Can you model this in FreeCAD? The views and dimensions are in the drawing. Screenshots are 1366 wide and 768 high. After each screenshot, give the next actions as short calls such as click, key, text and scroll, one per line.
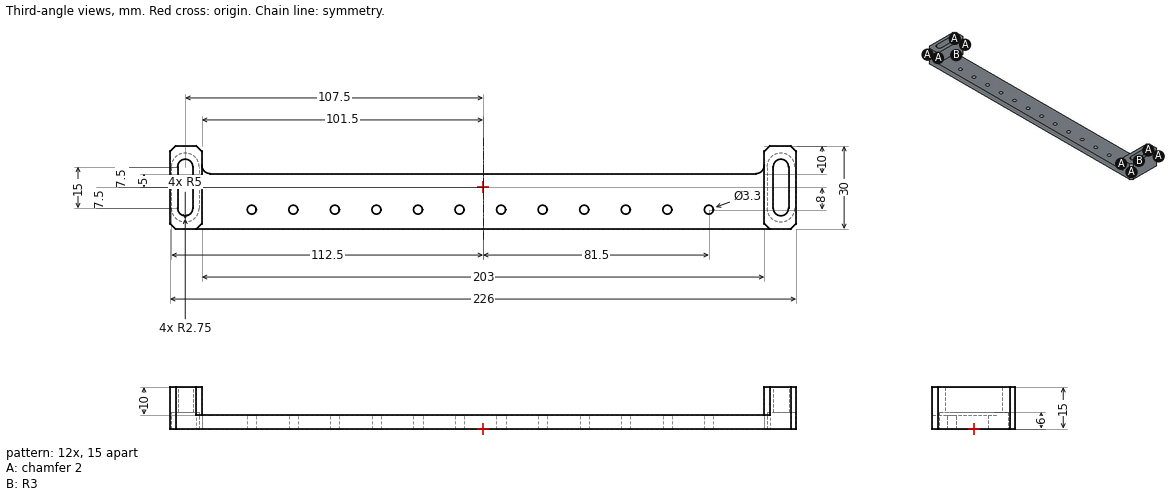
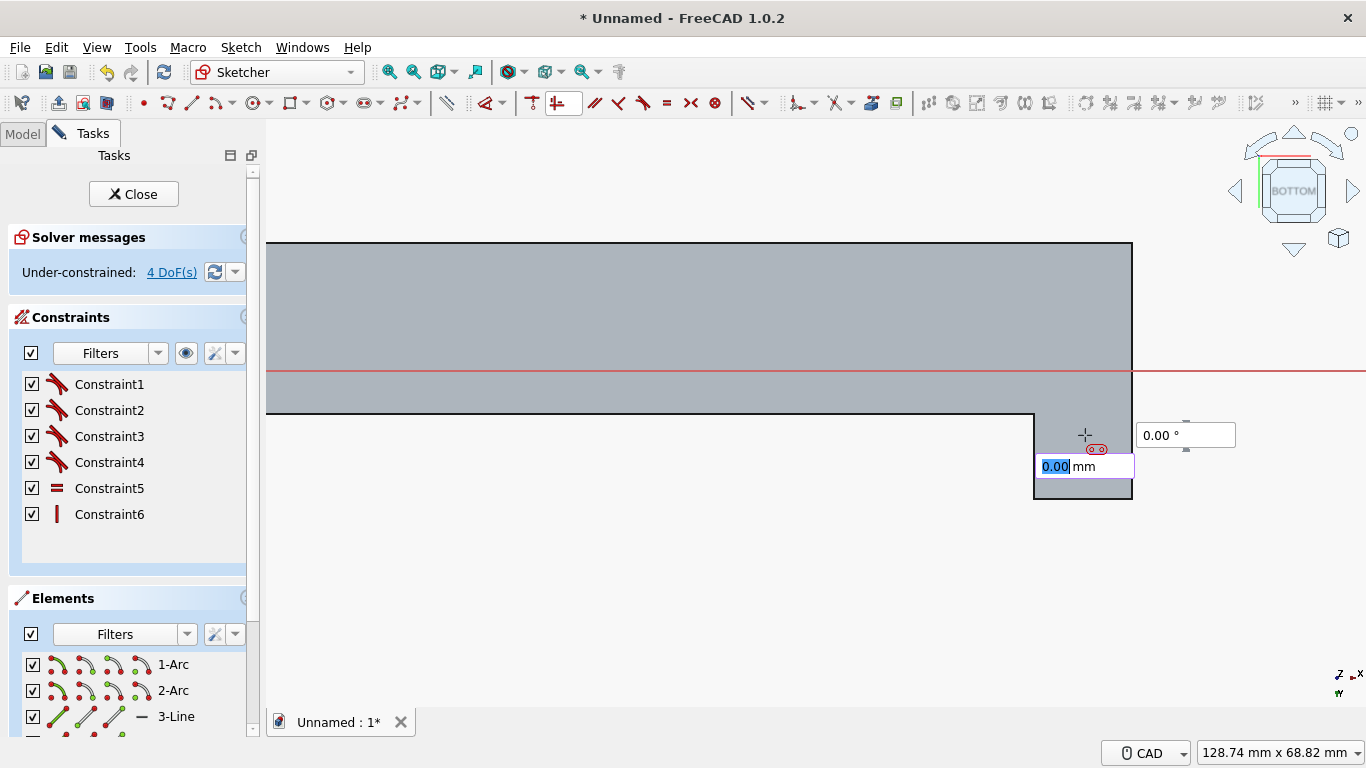
click(1085, 307)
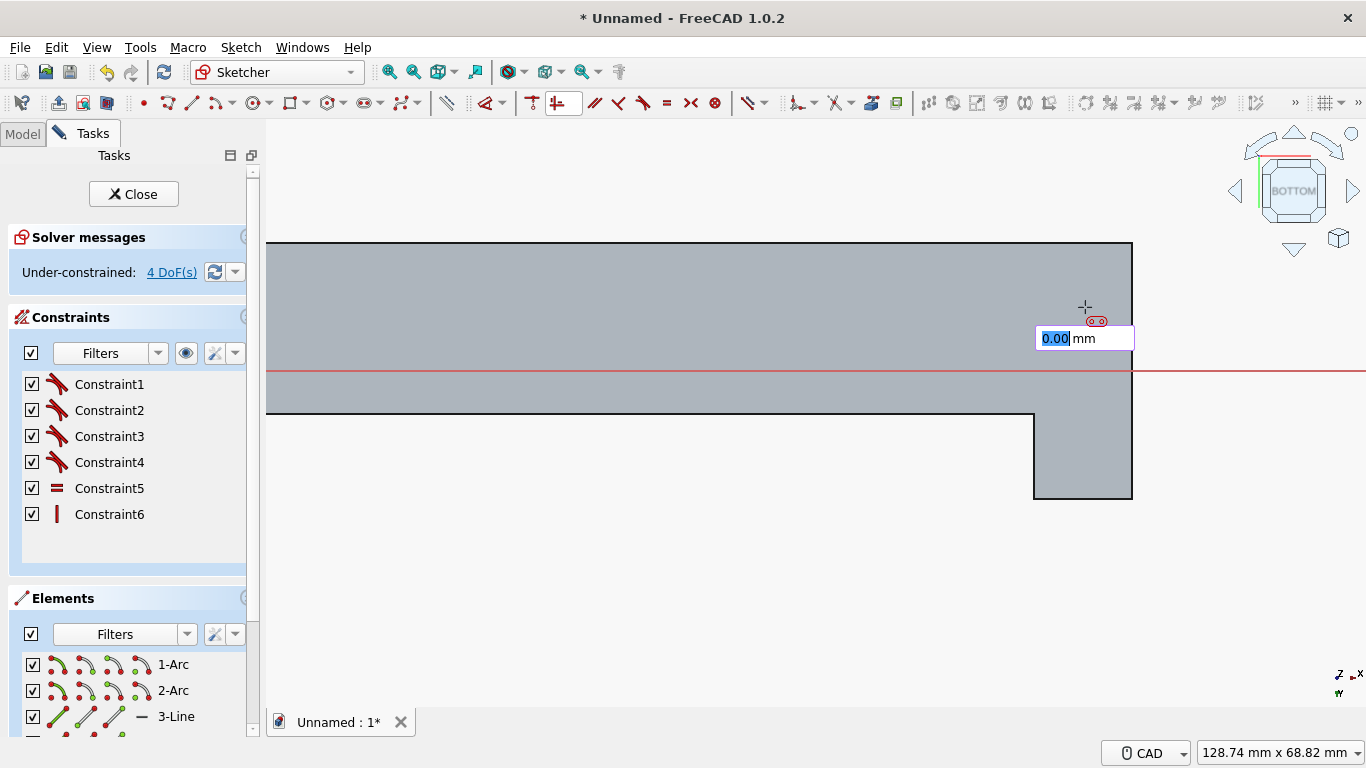
click(1109, 390)
key(Escape)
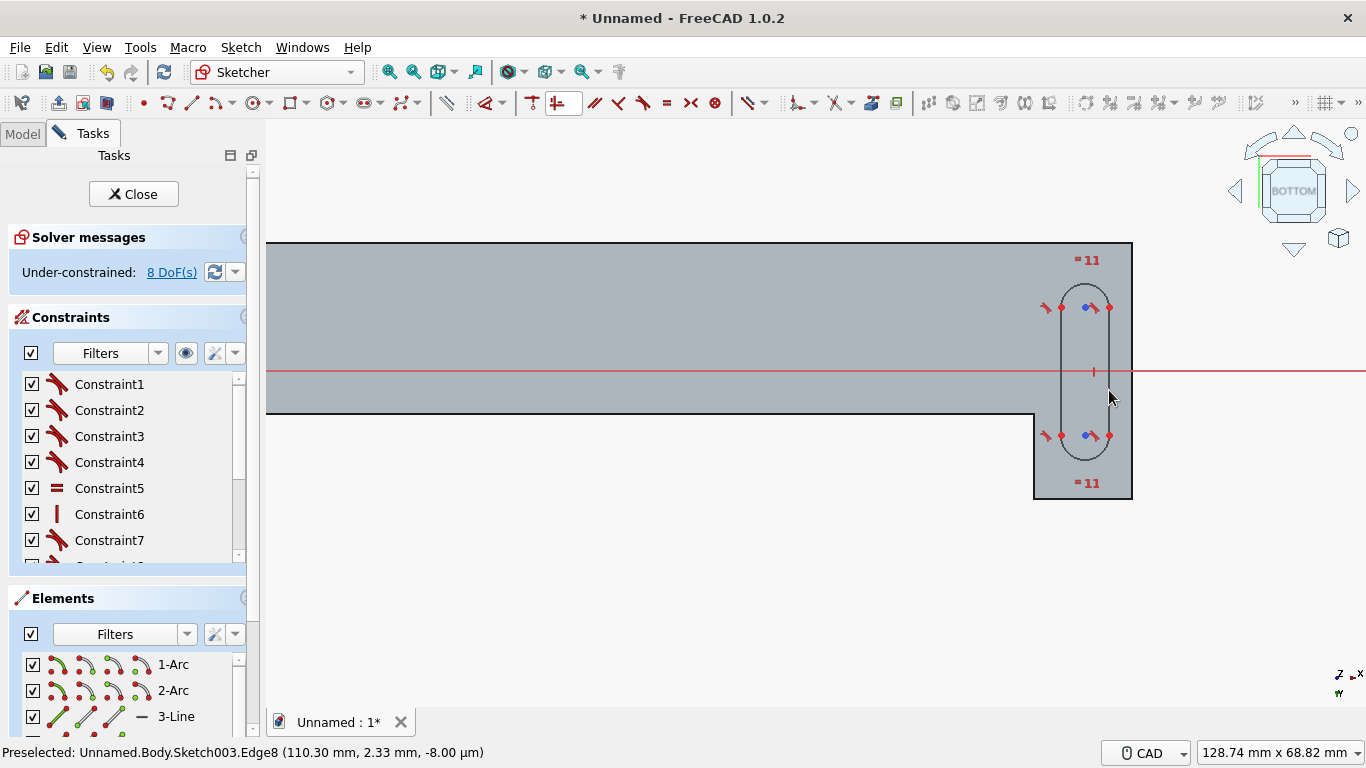
scroll(1086, 437, down, 5)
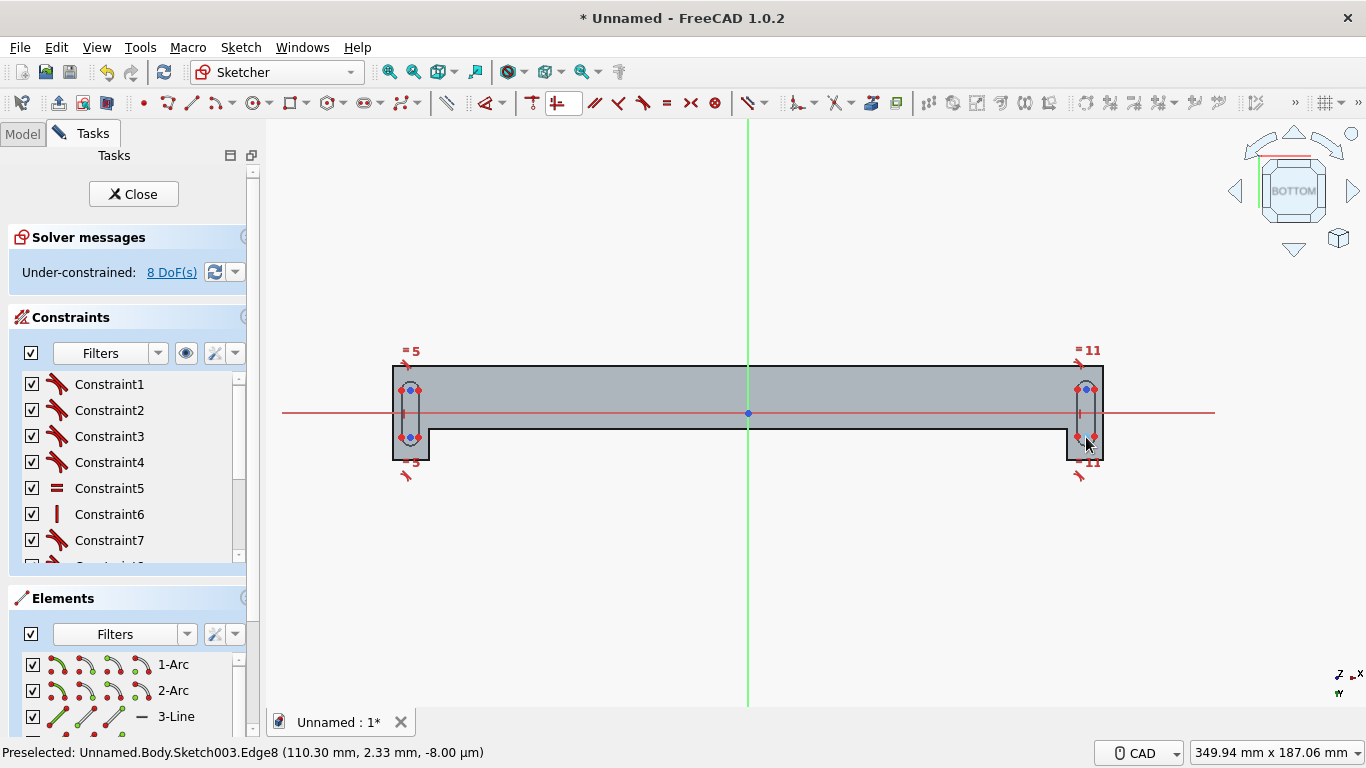
scroll(405, 444, up, 3)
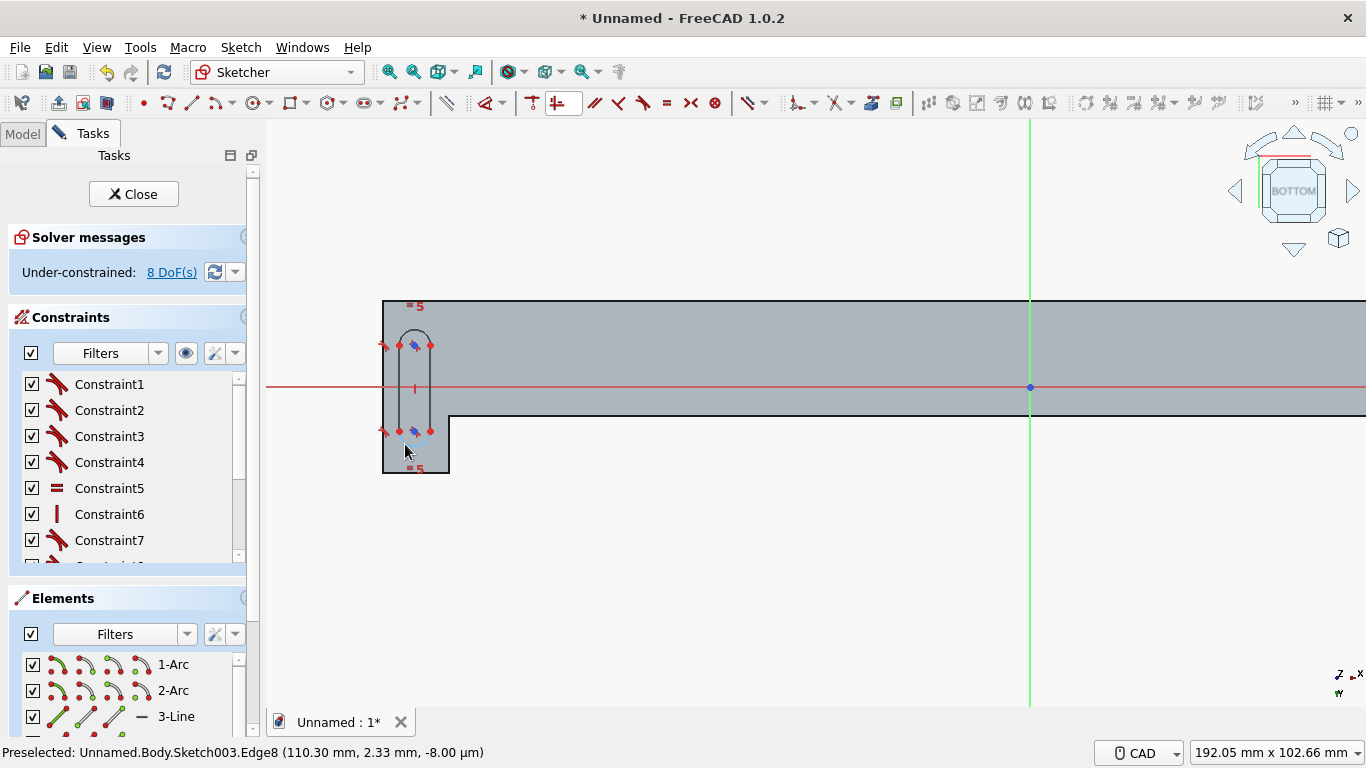
click(406, 444)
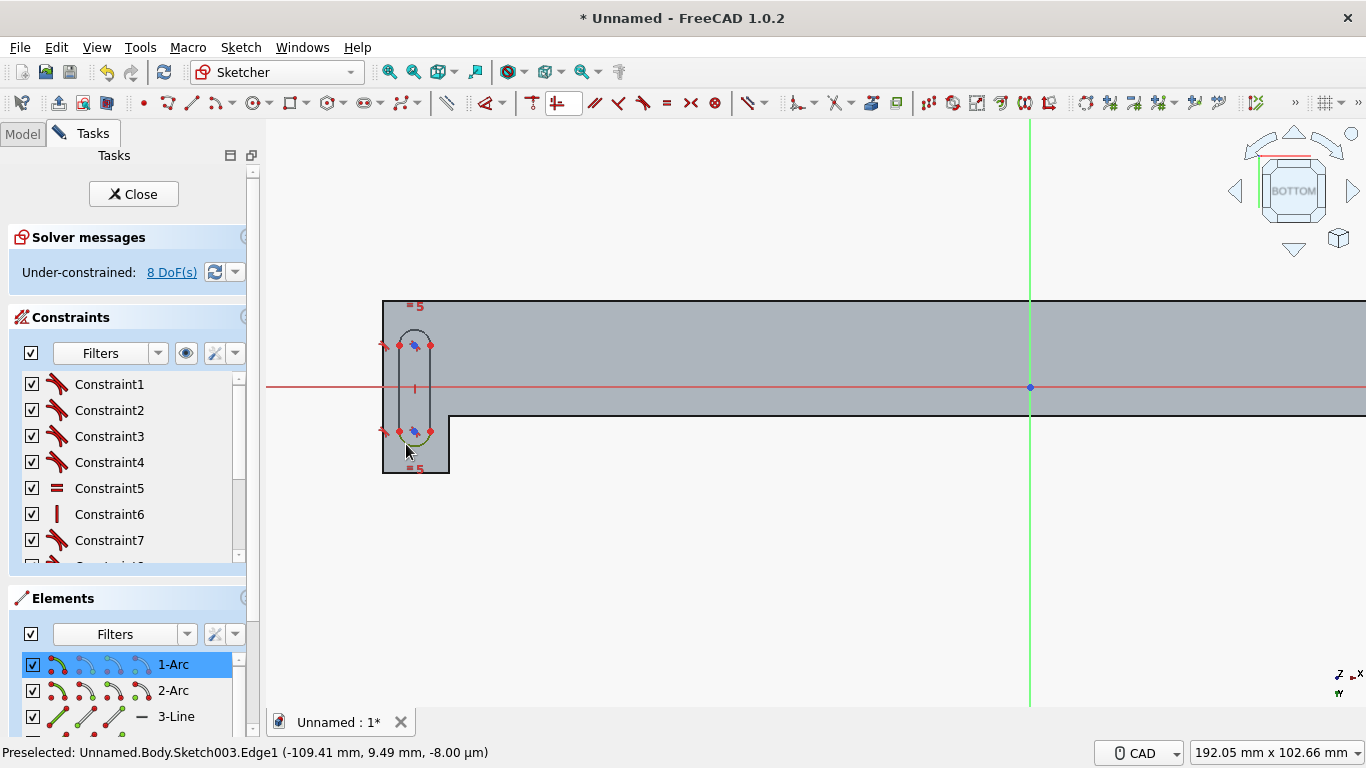
scroll(404, 444, down, 3)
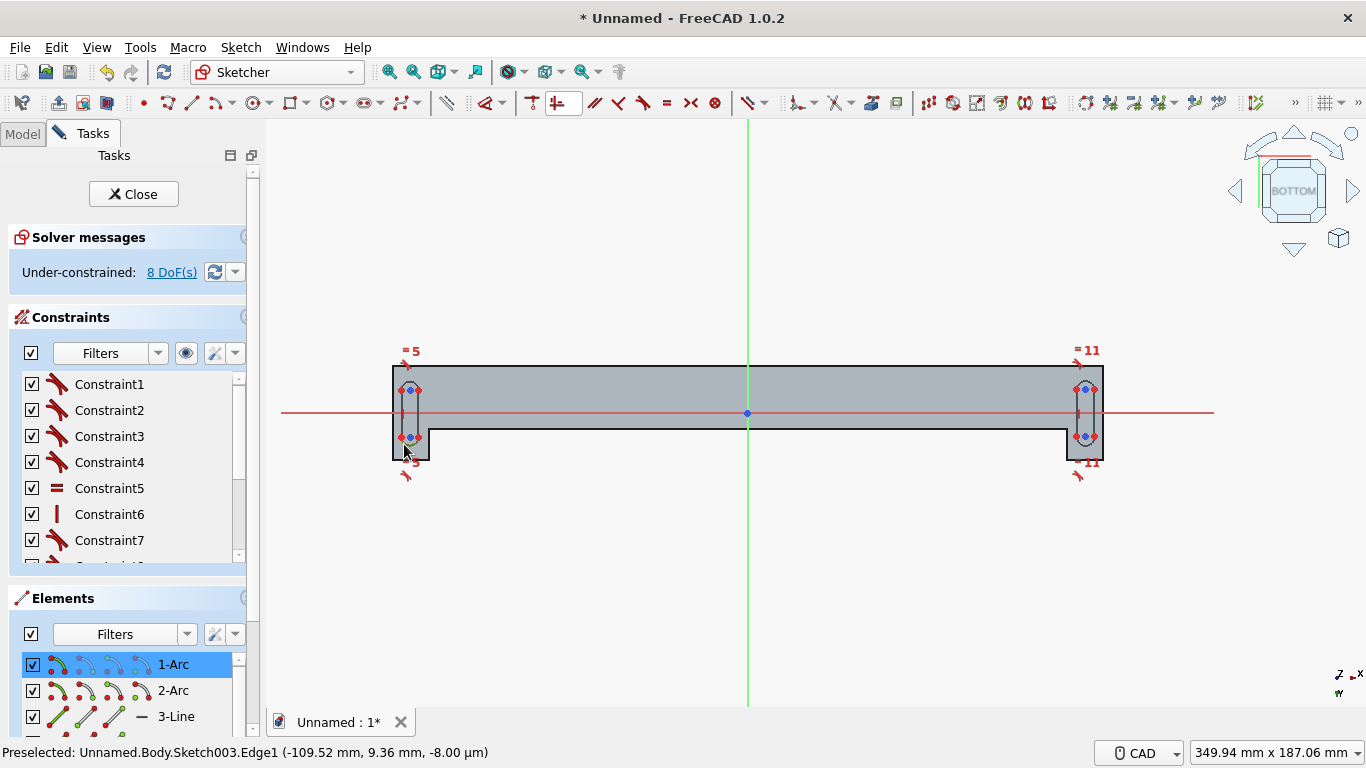
scroll(1080, 444, up, 3)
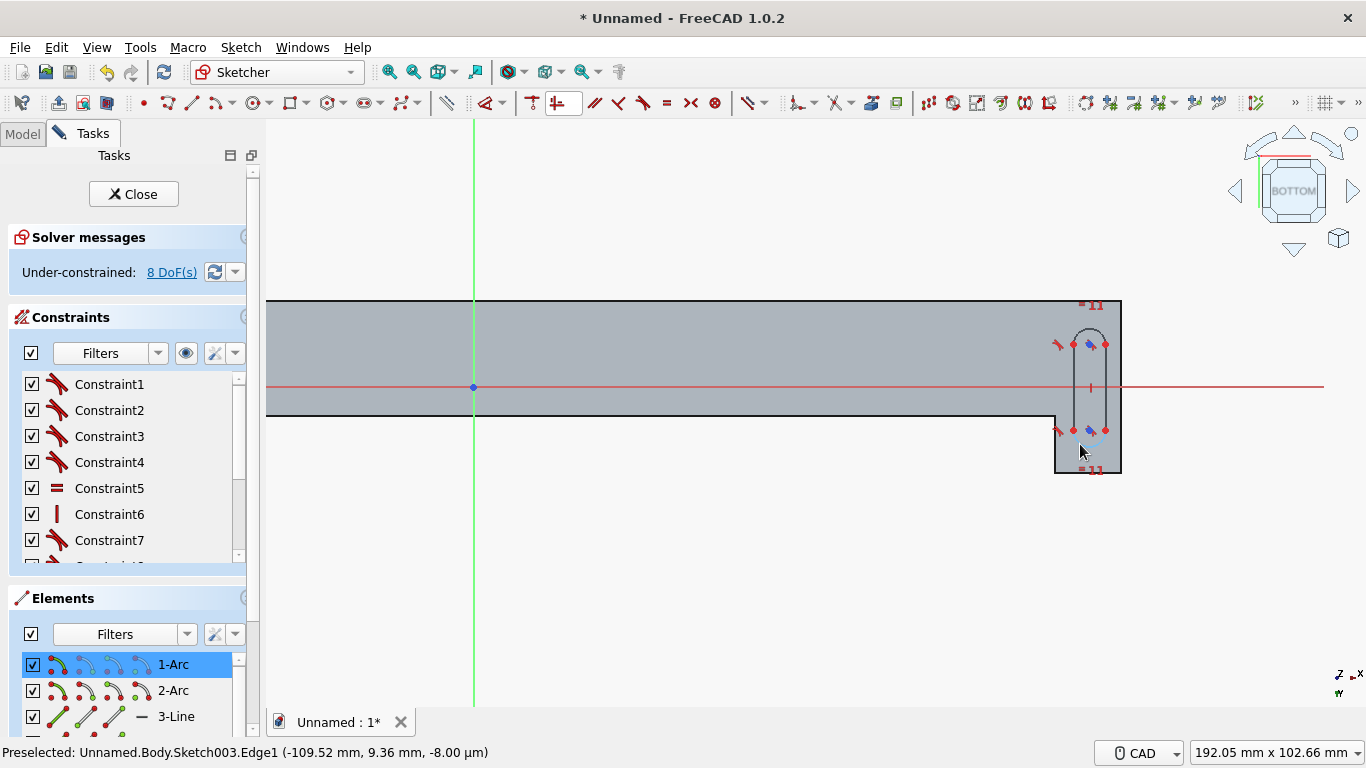
click(1080, 444)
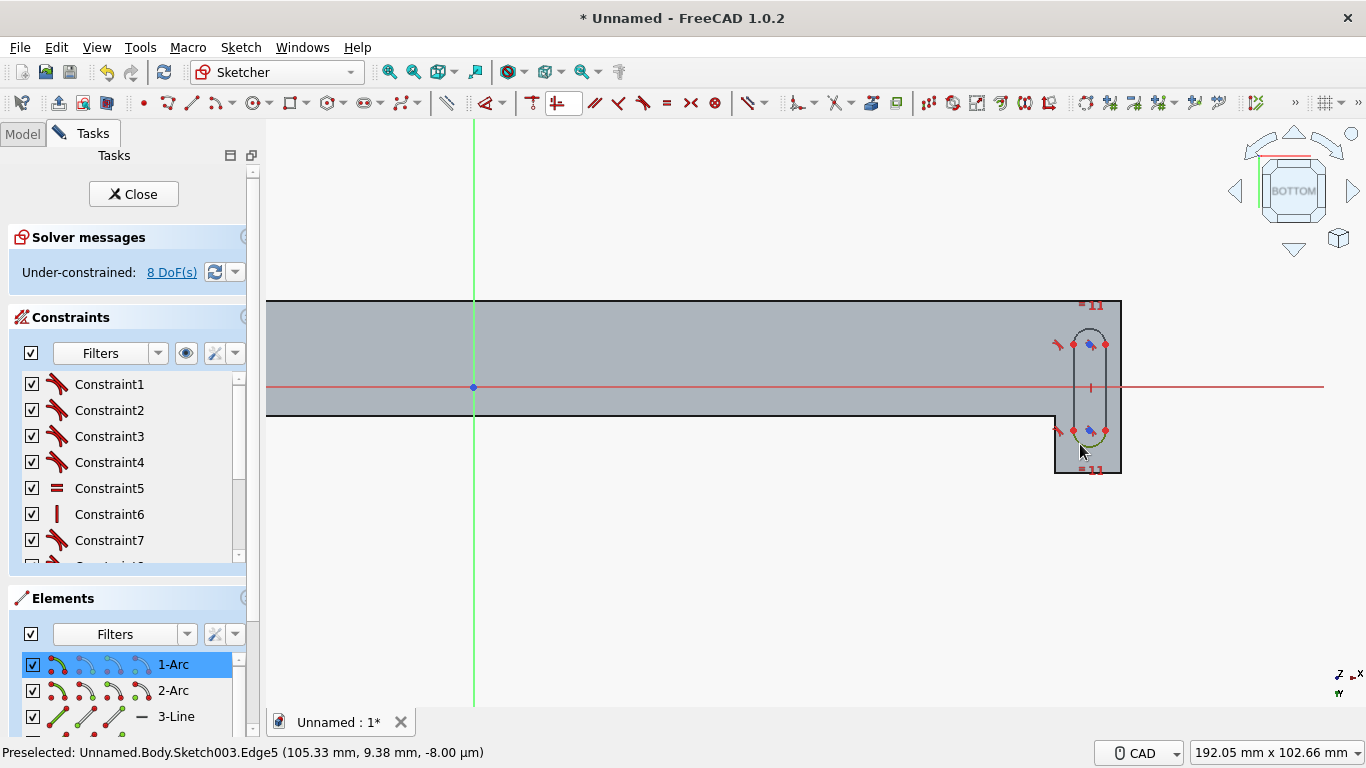
click(668, 104)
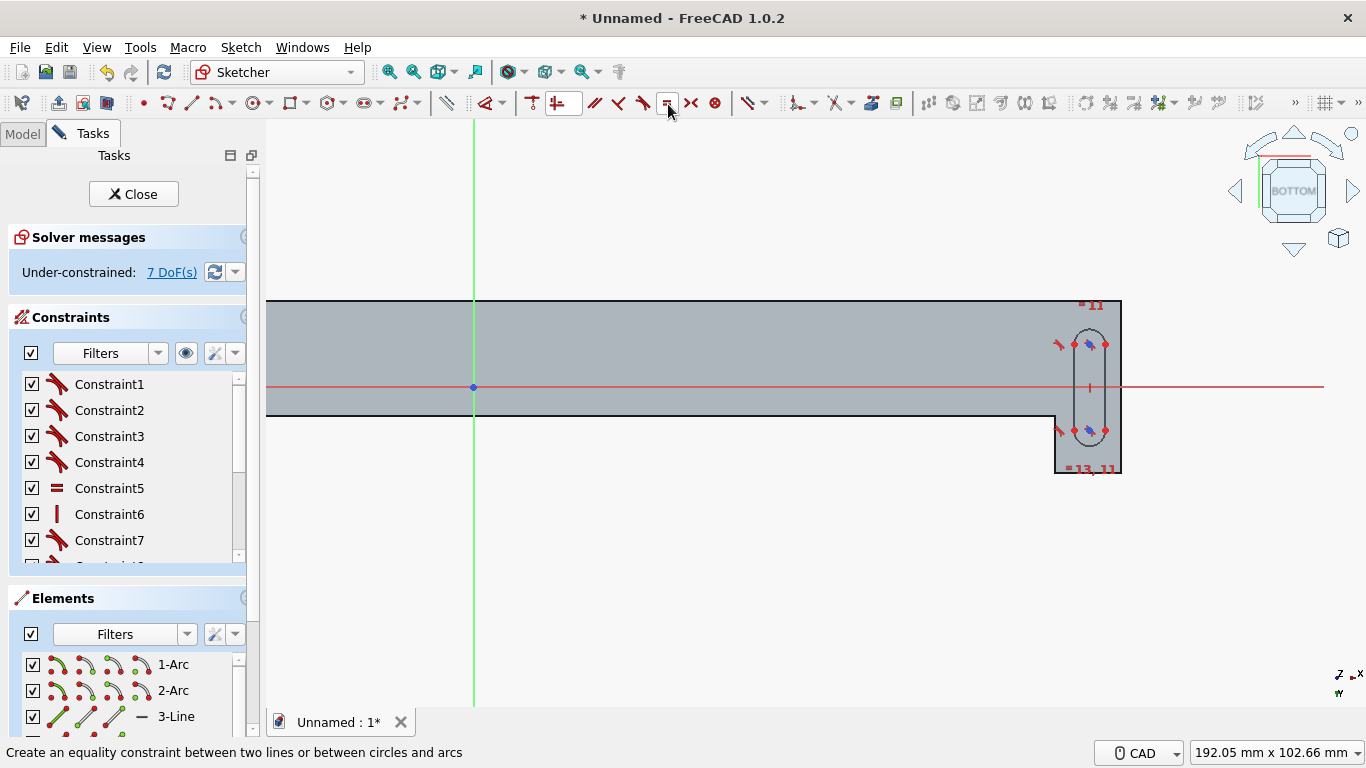
scroll(1080, 444, down, 3)